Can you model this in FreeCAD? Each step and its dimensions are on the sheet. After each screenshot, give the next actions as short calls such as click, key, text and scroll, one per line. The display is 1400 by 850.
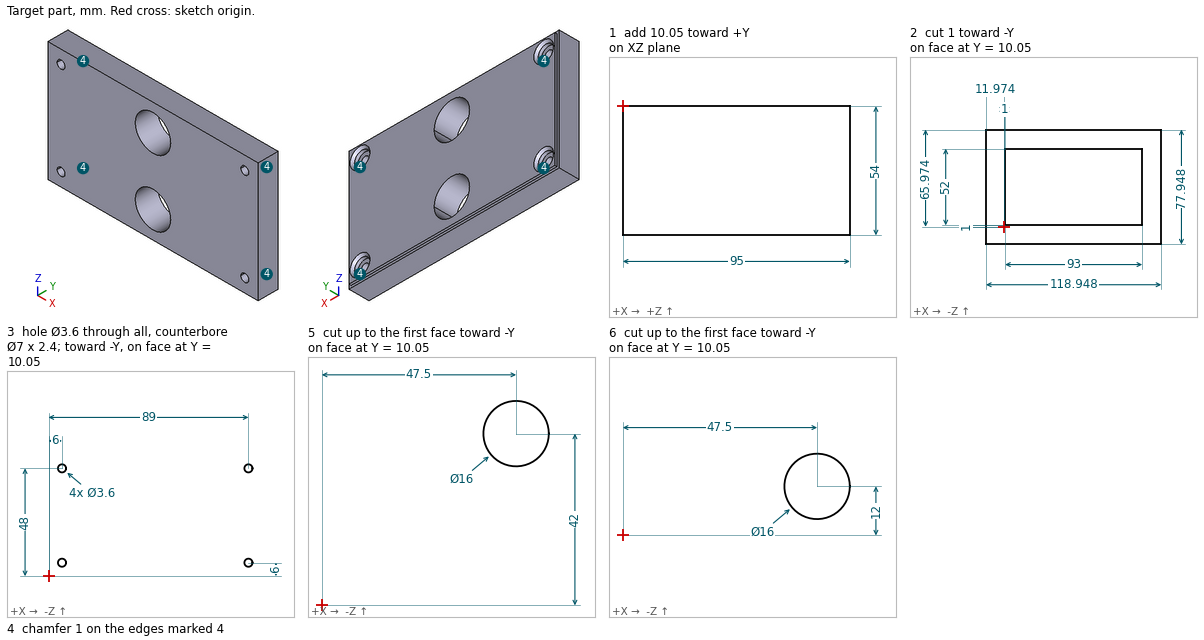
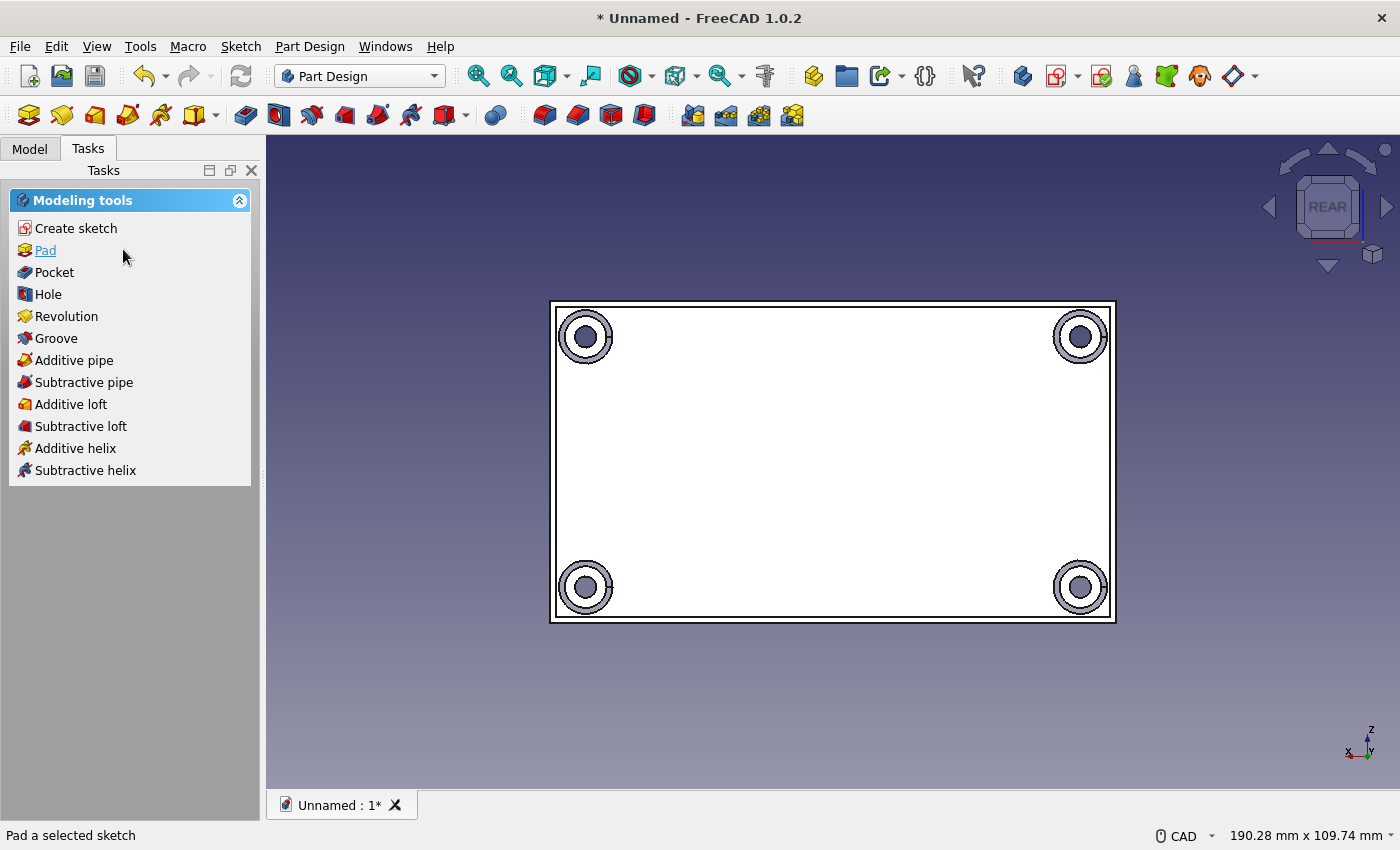
click(246, 116)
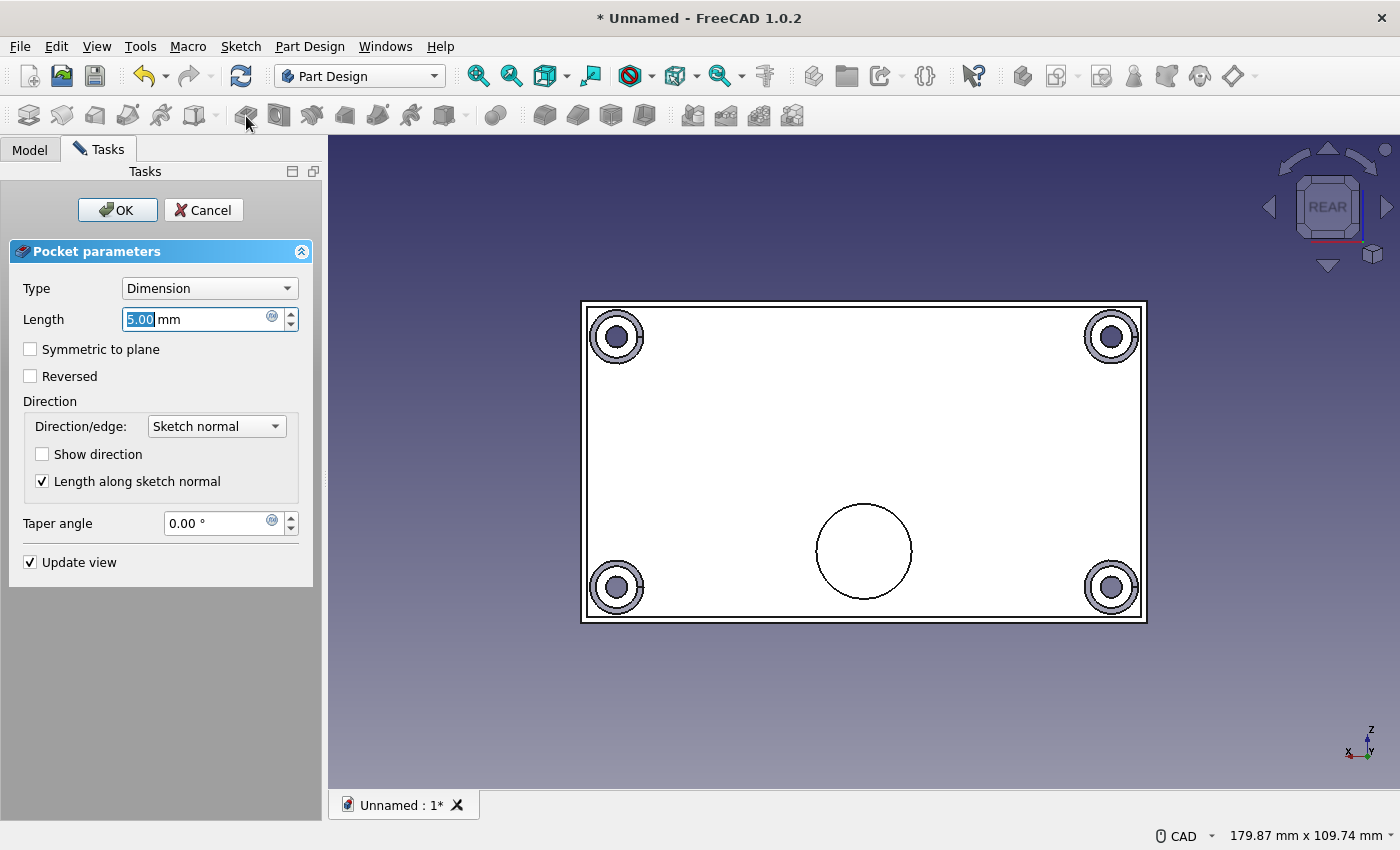
click(210, 288)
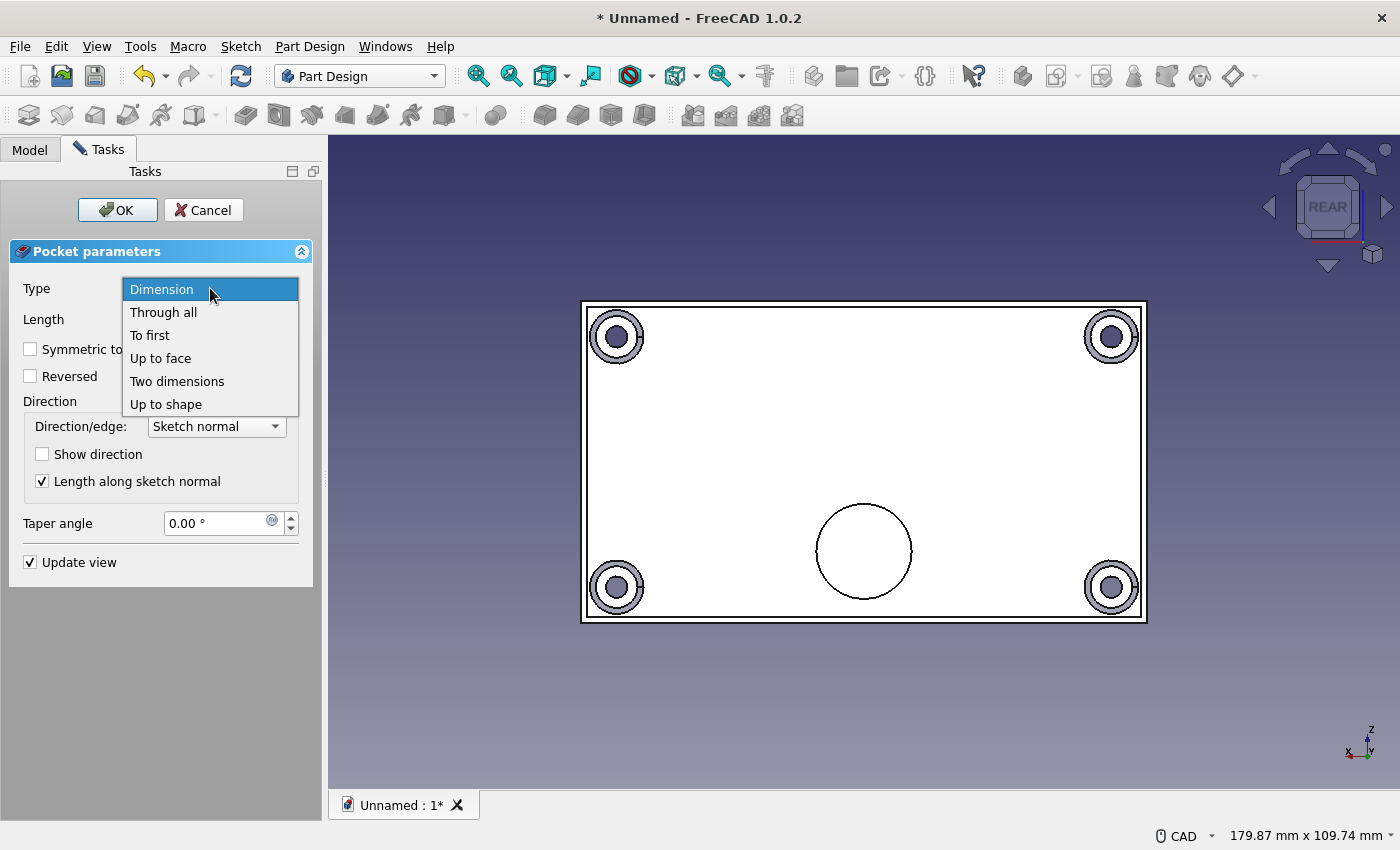
click(208, 336)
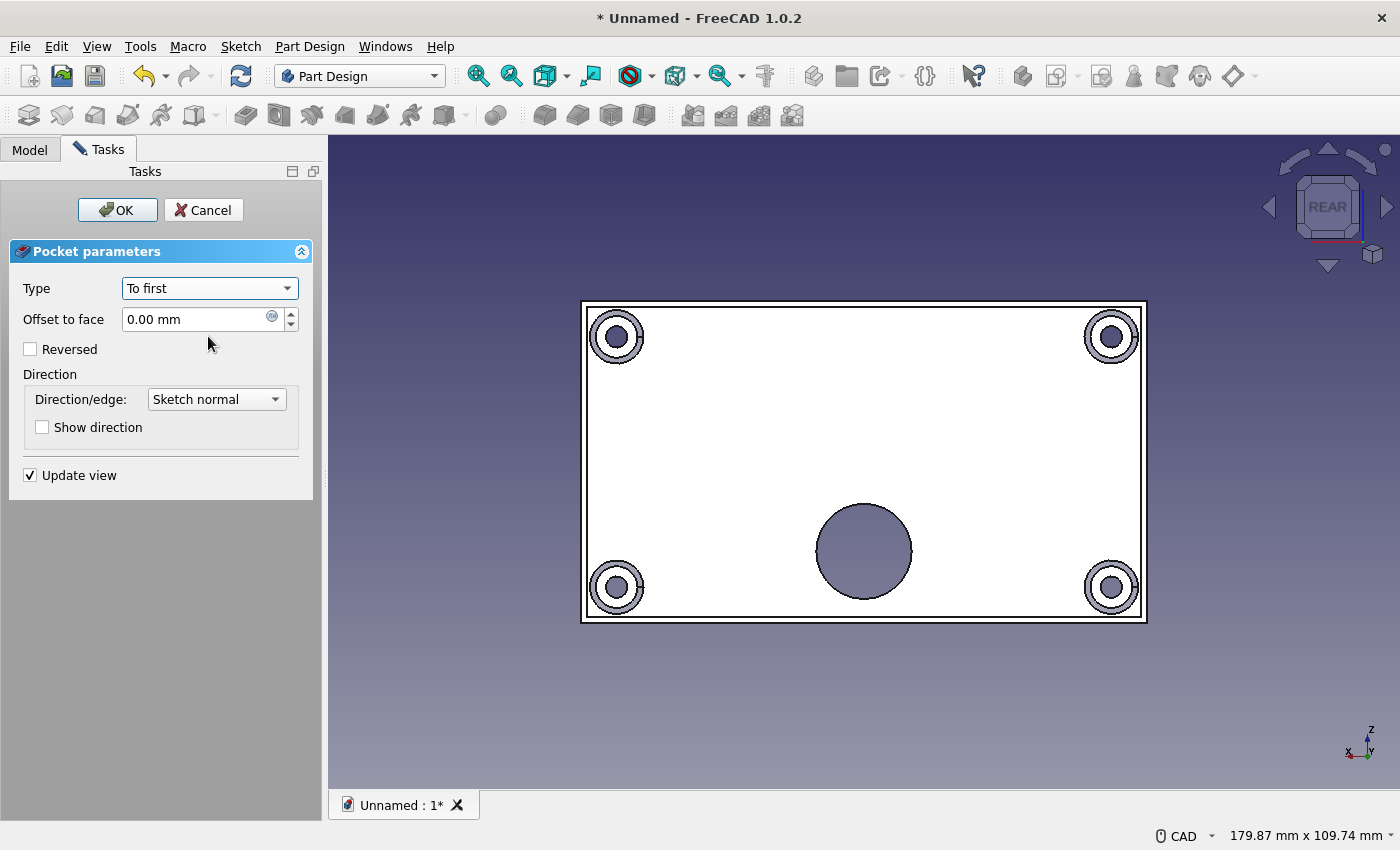
click(118, 210)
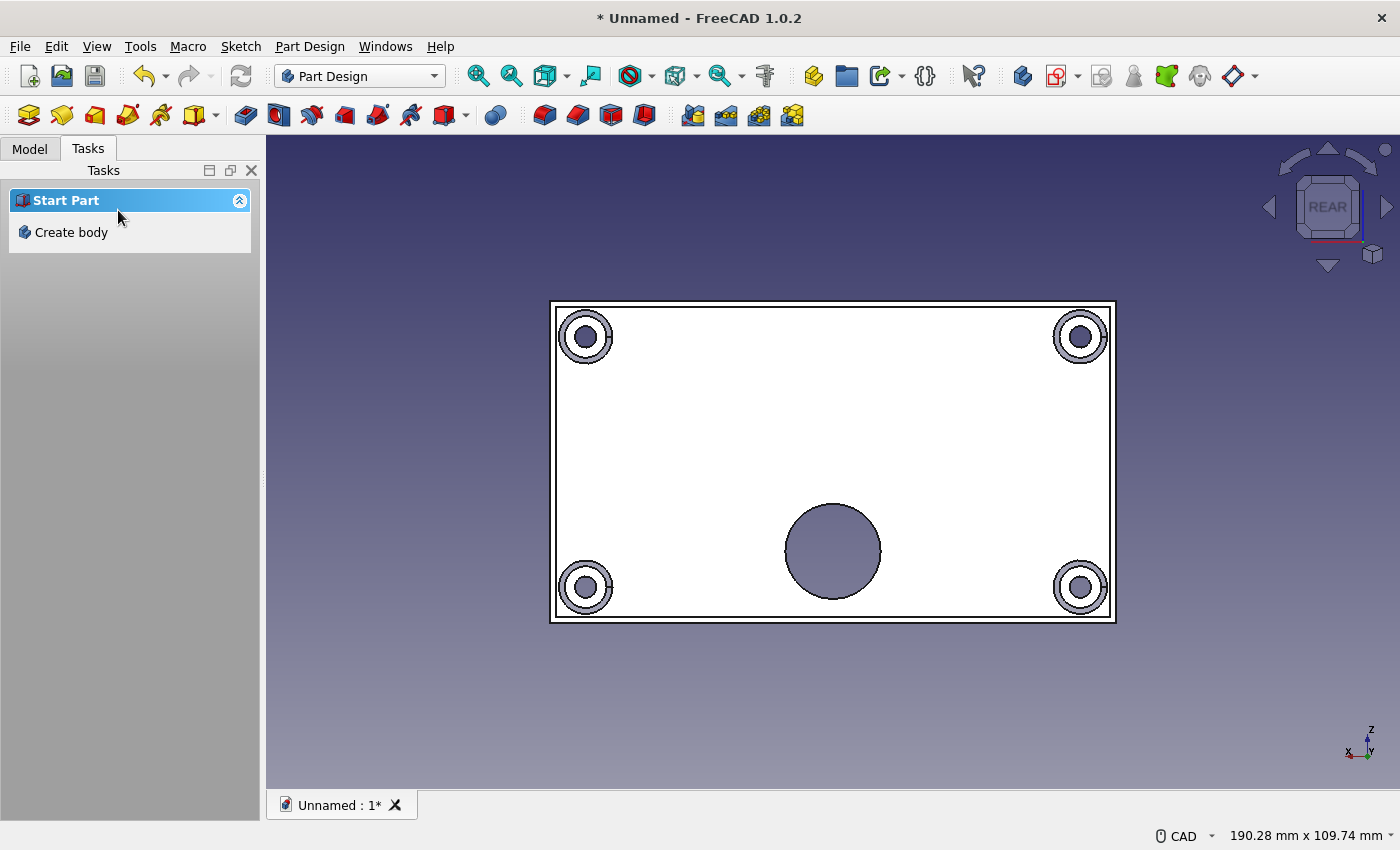
click(991, 461)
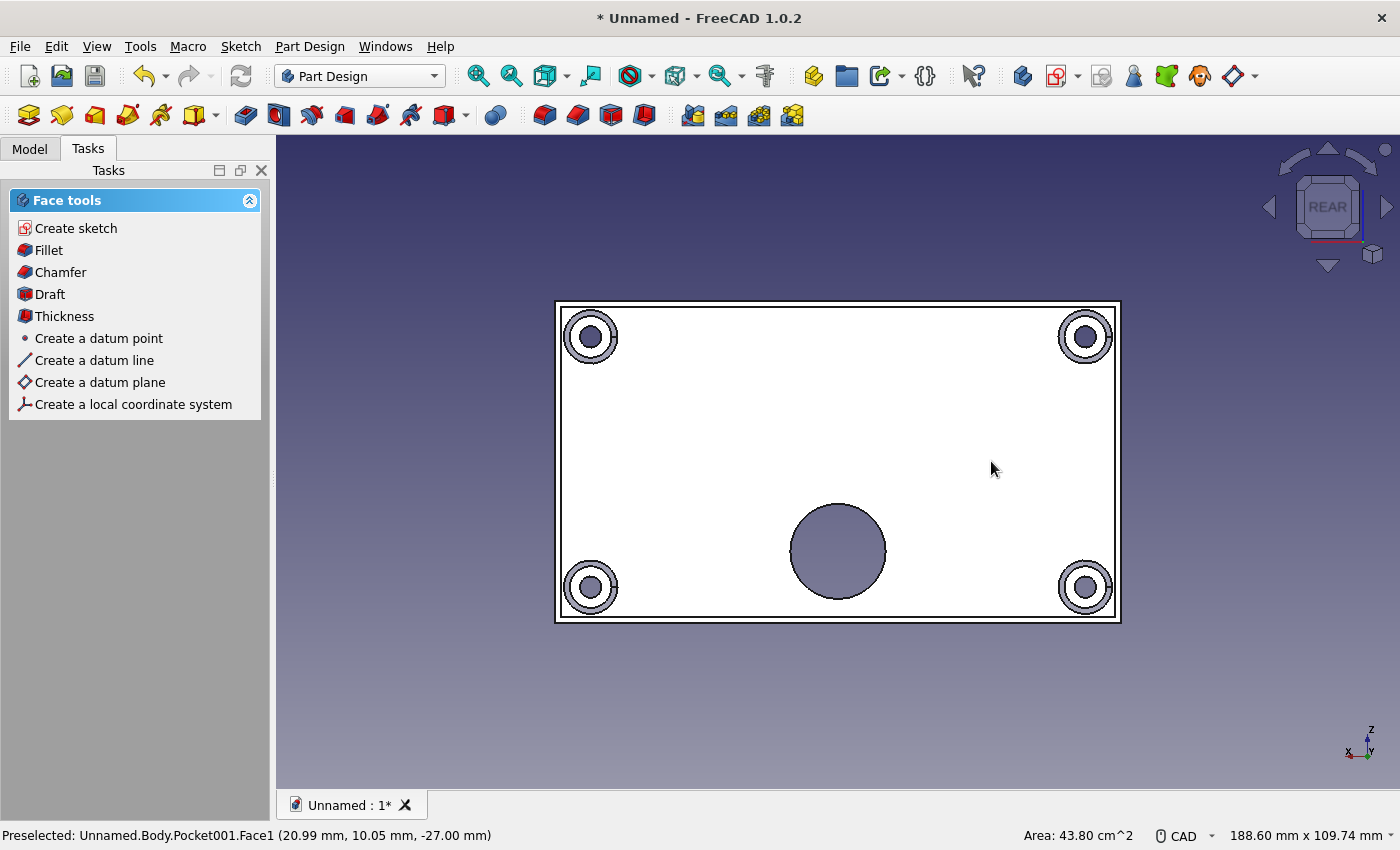
click(1056, 76)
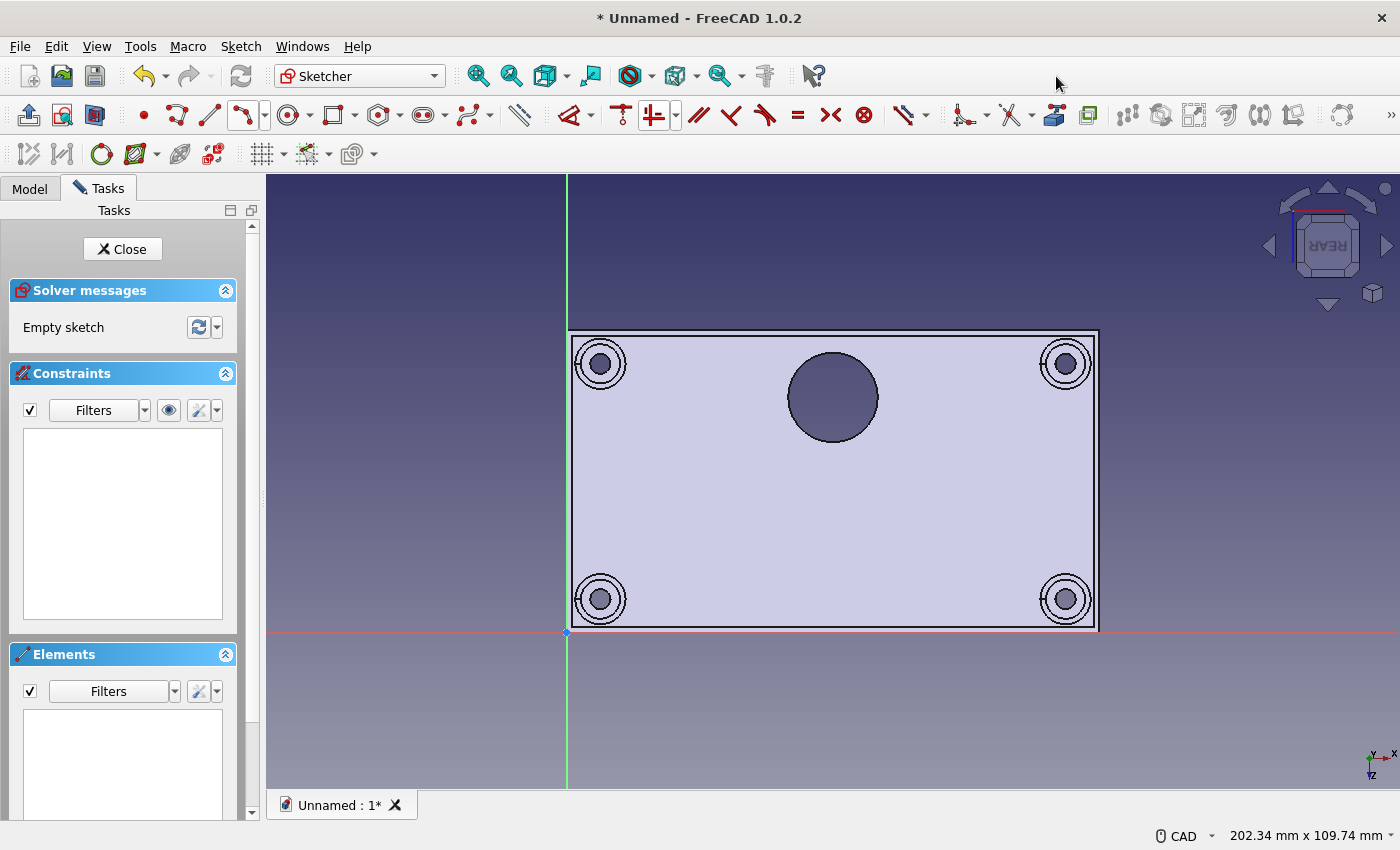
scroll(855, 593, up, 7)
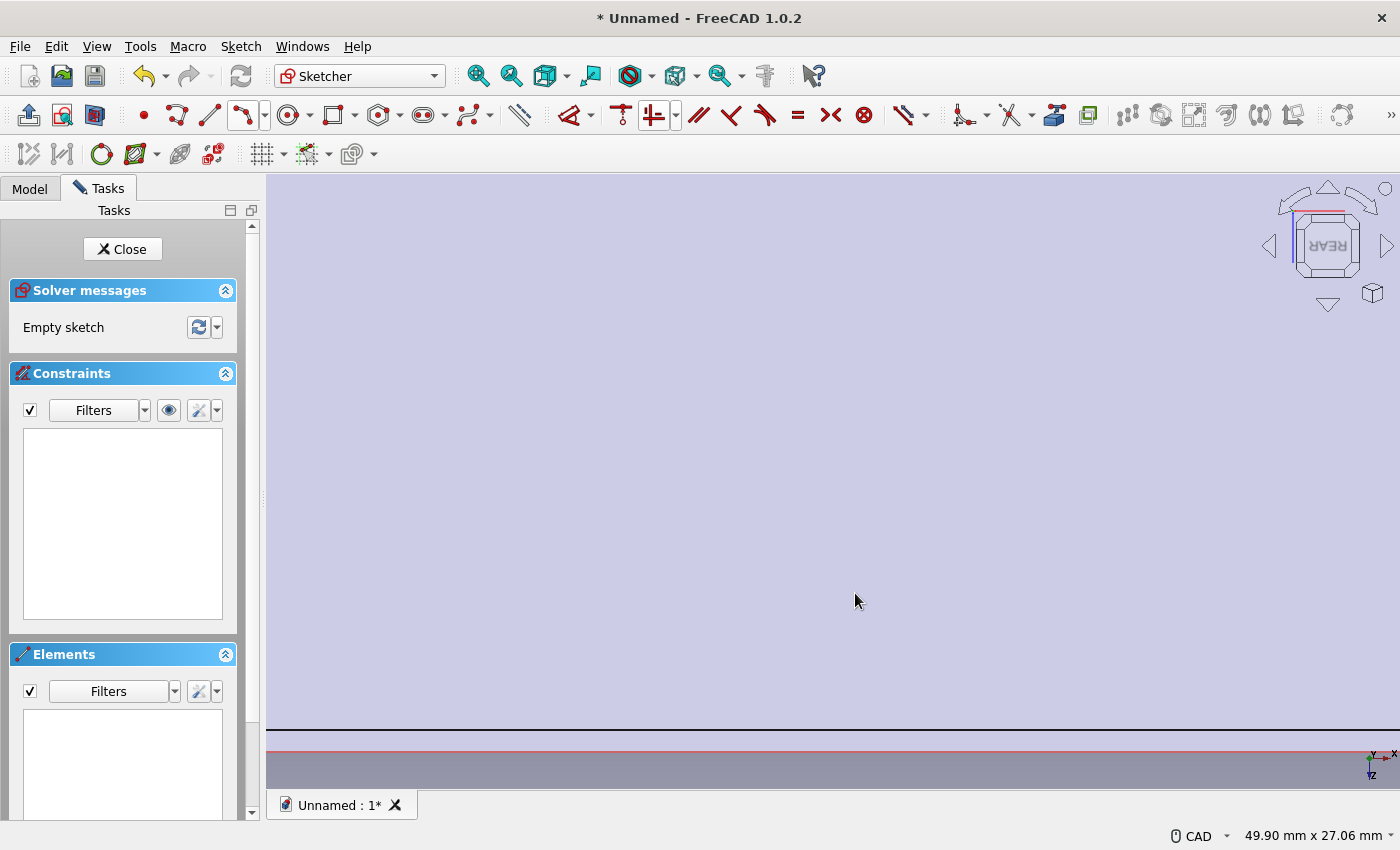
click(288, 116)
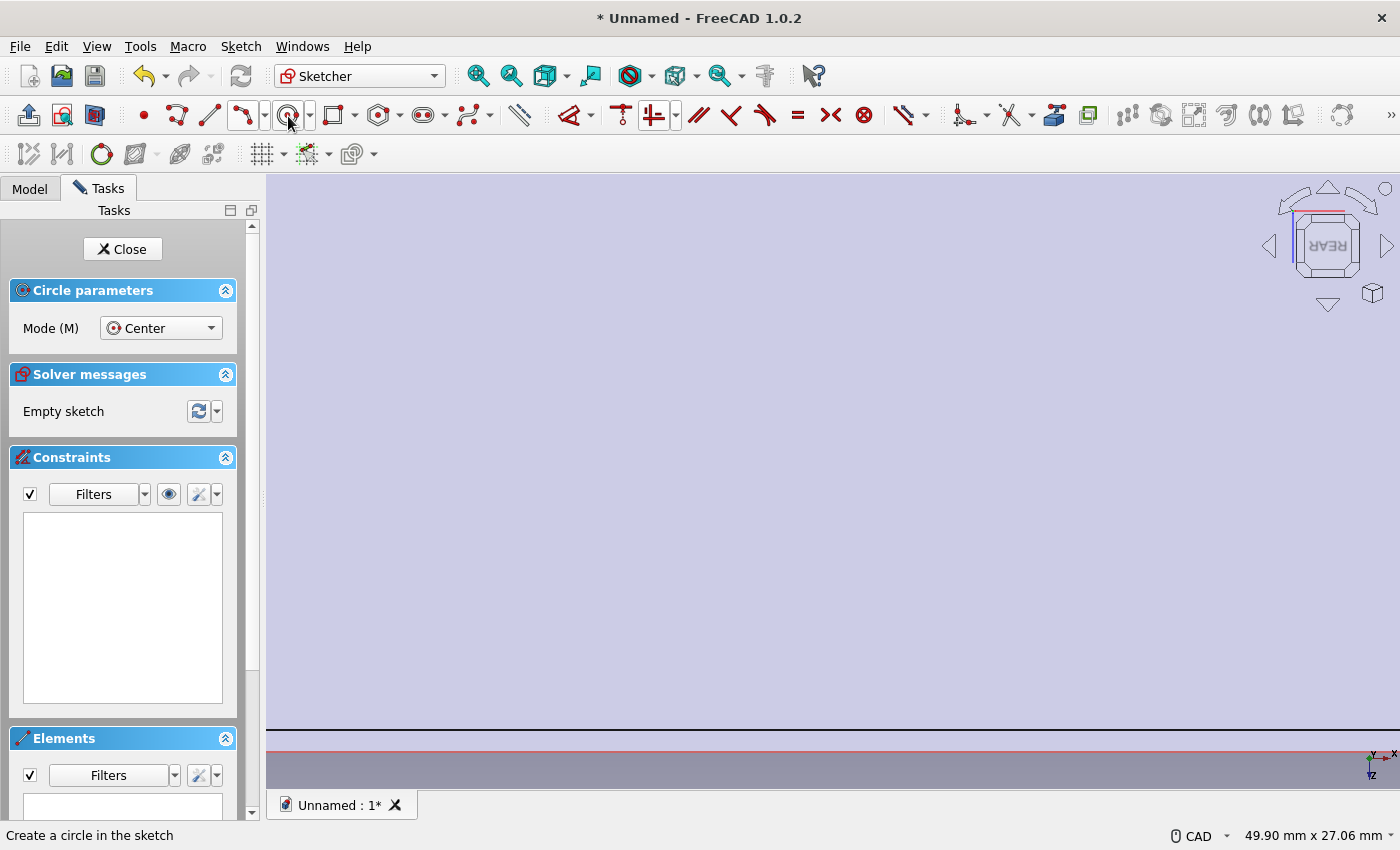
click(764, 480)
move(893, 351)